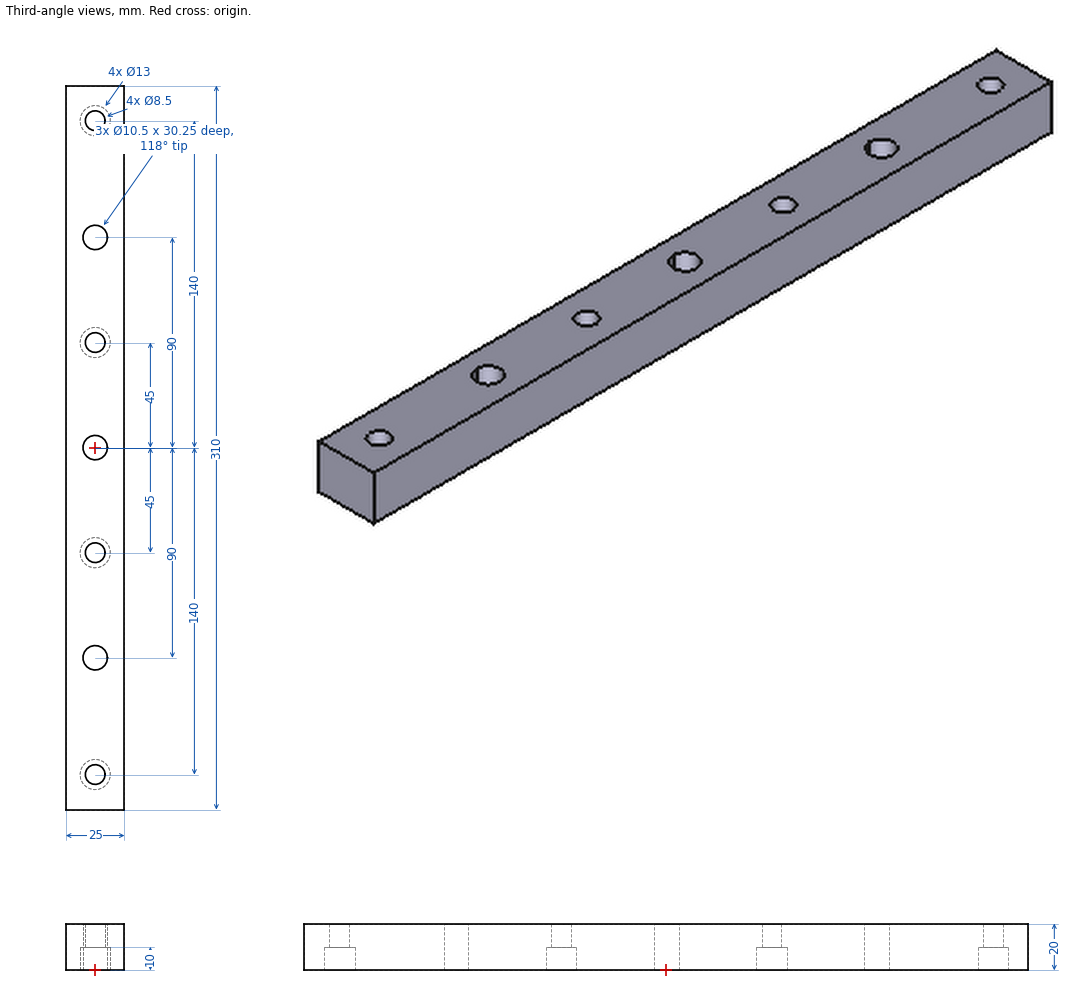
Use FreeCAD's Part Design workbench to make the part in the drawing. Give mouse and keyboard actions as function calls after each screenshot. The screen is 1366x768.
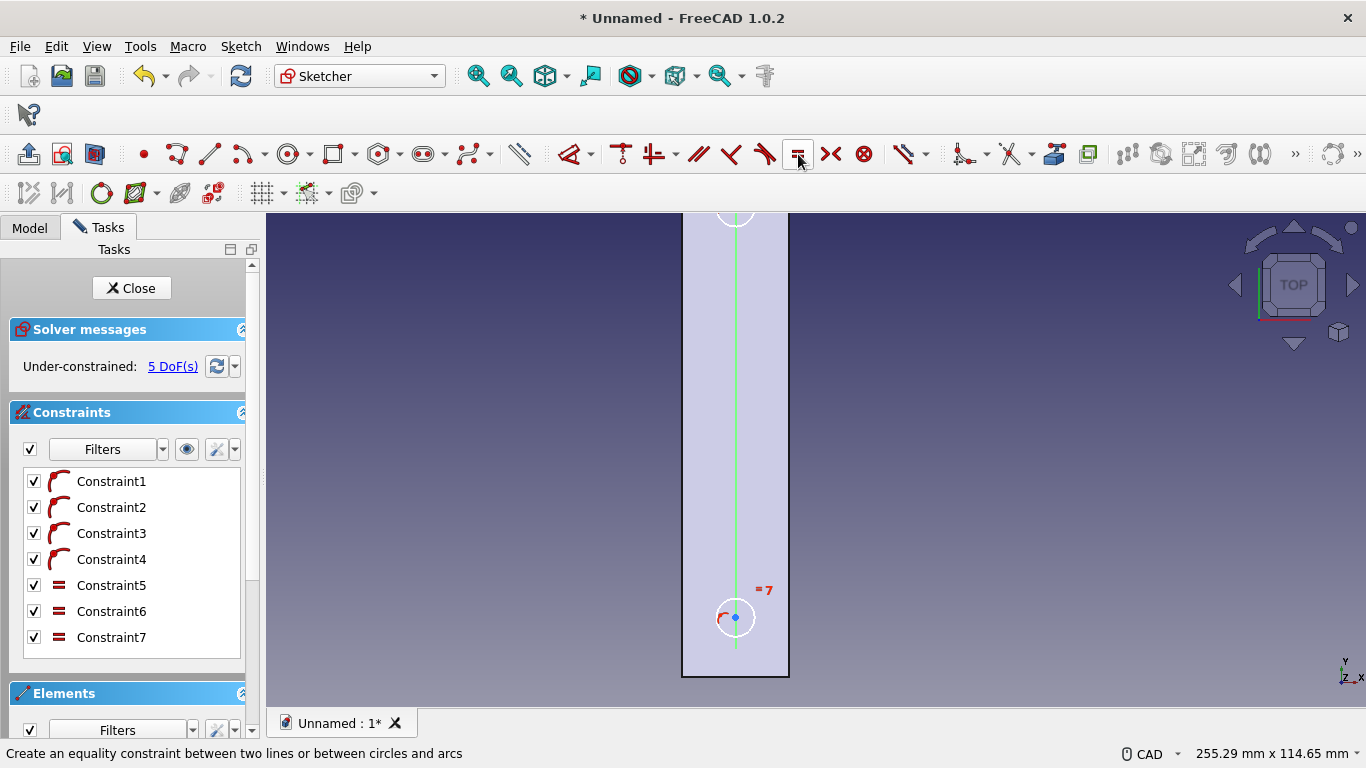
key(d)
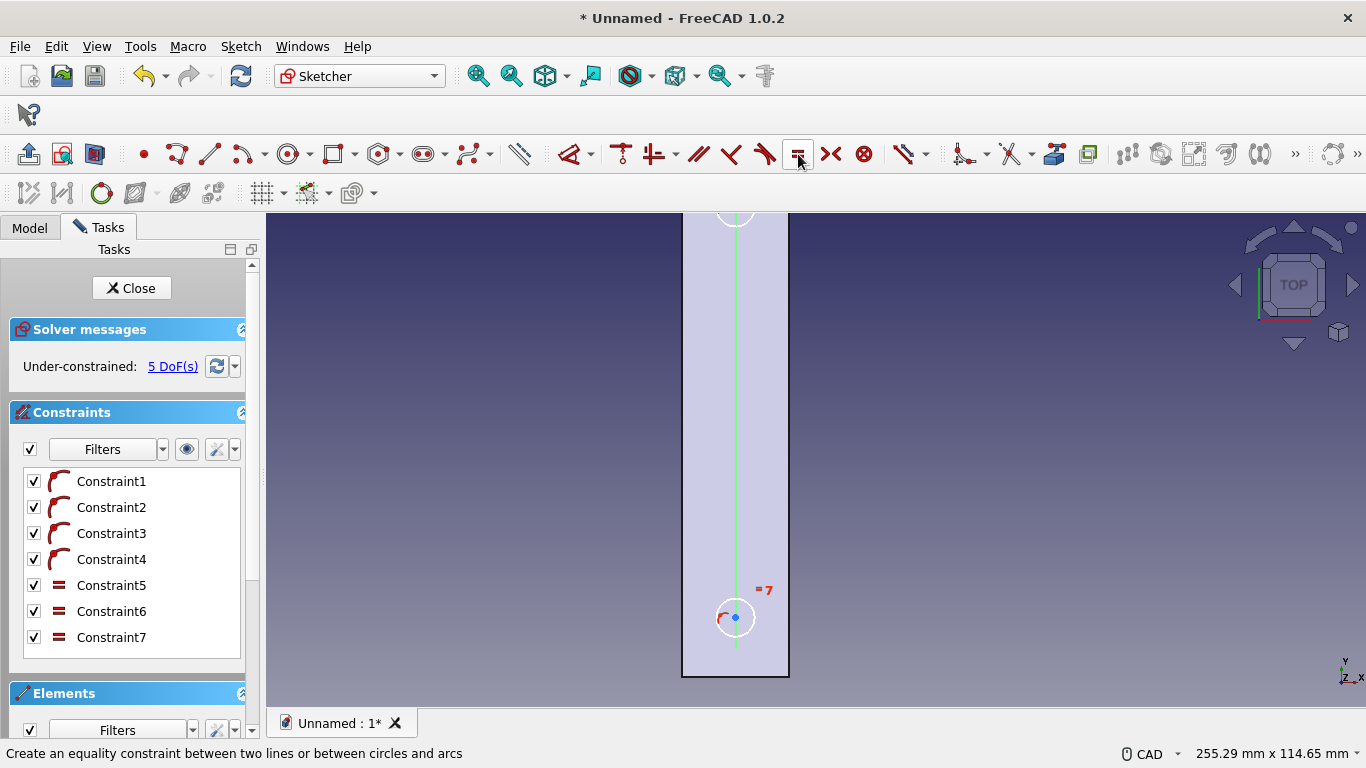
scroll(751, 607, down, 7)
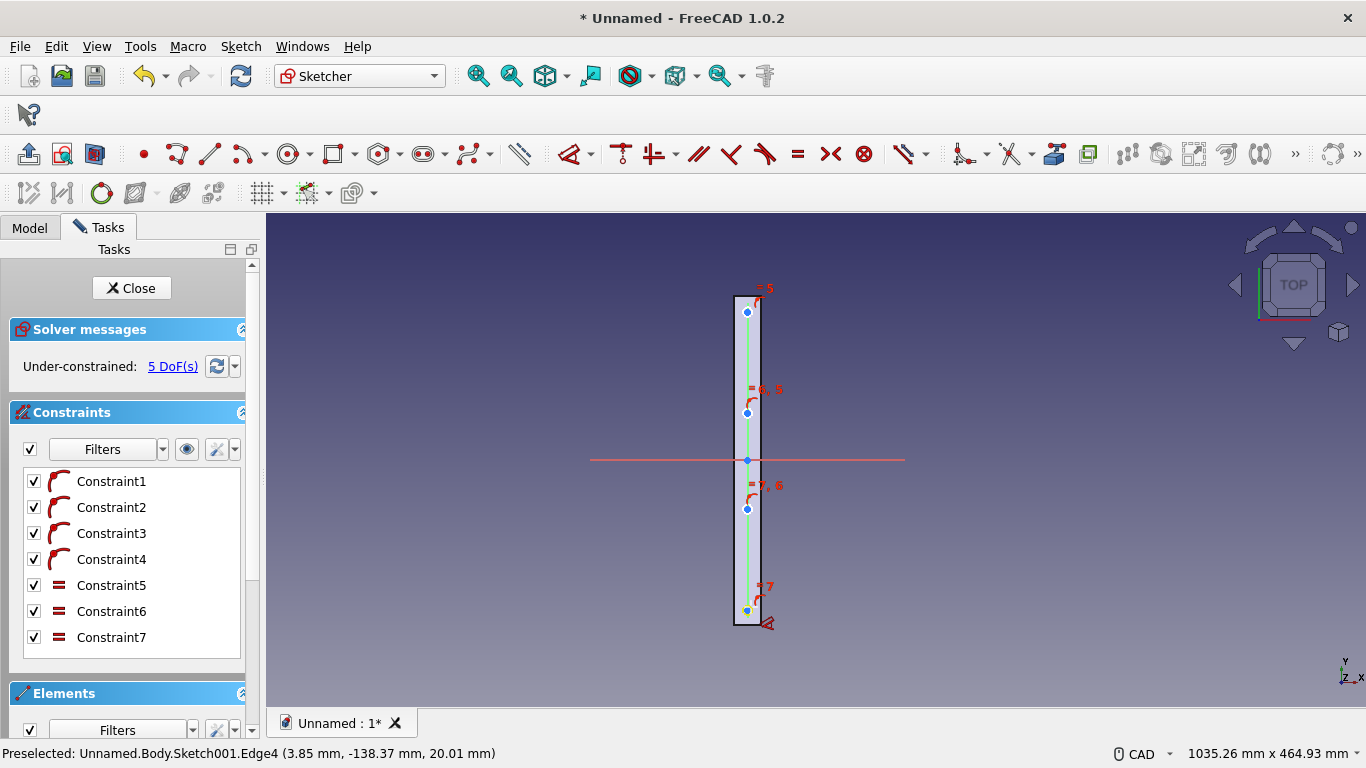
scroll(751, 309, up, 8)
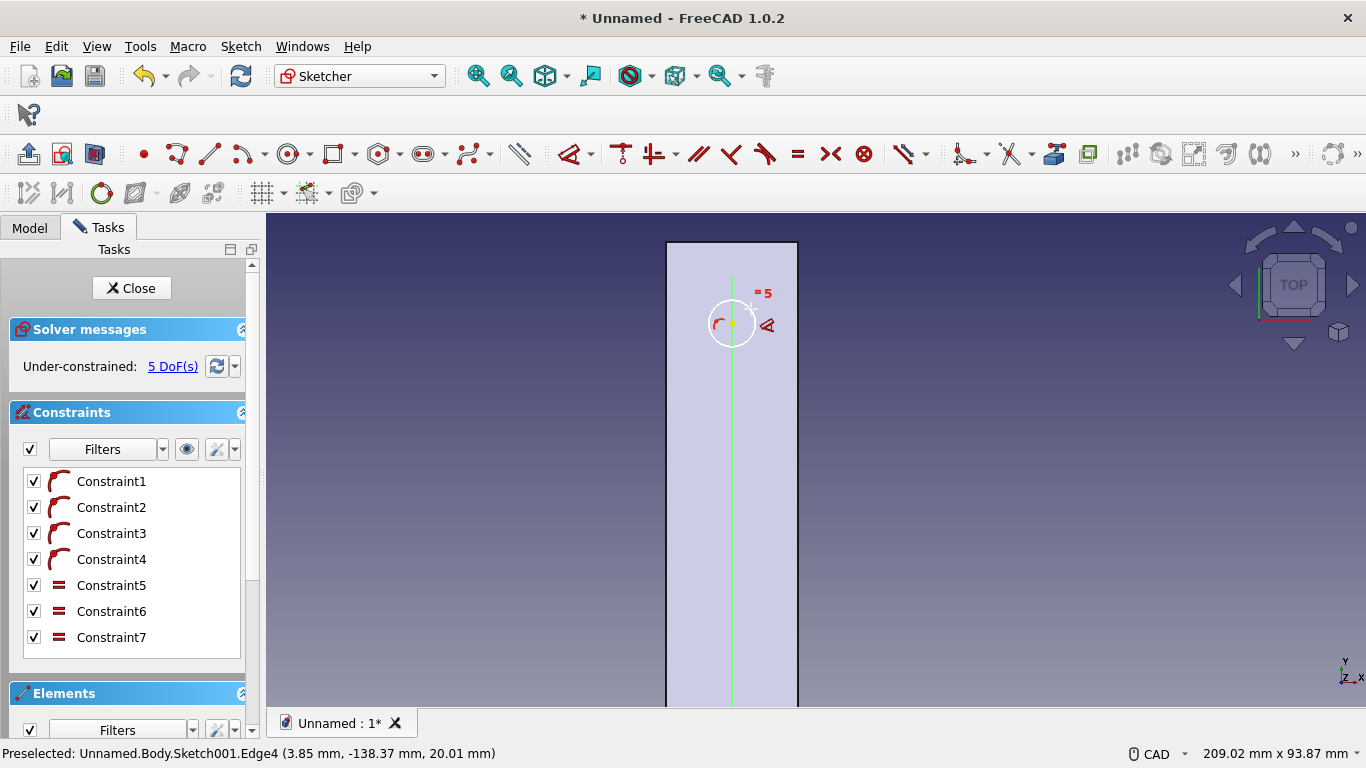
click(748, 307)
click(770, 284)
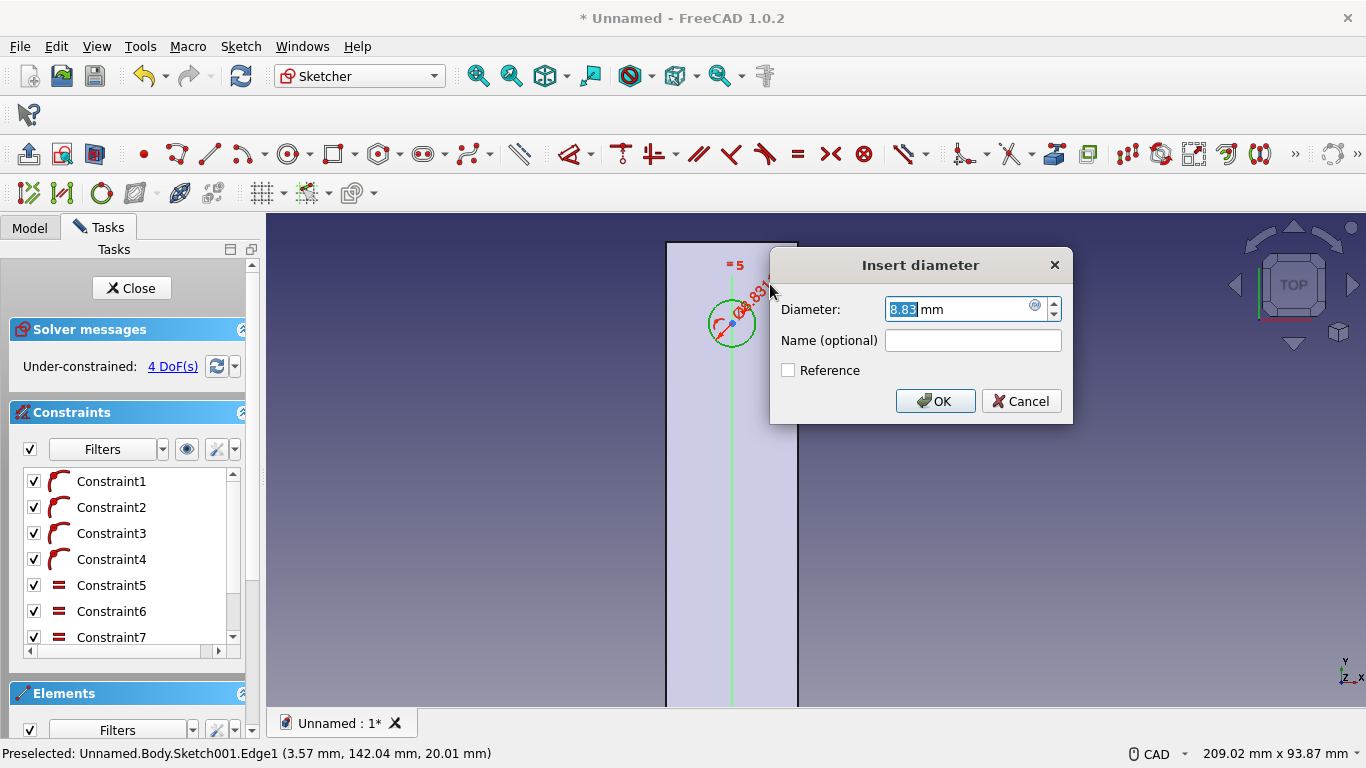
text(8.5)
key(Return)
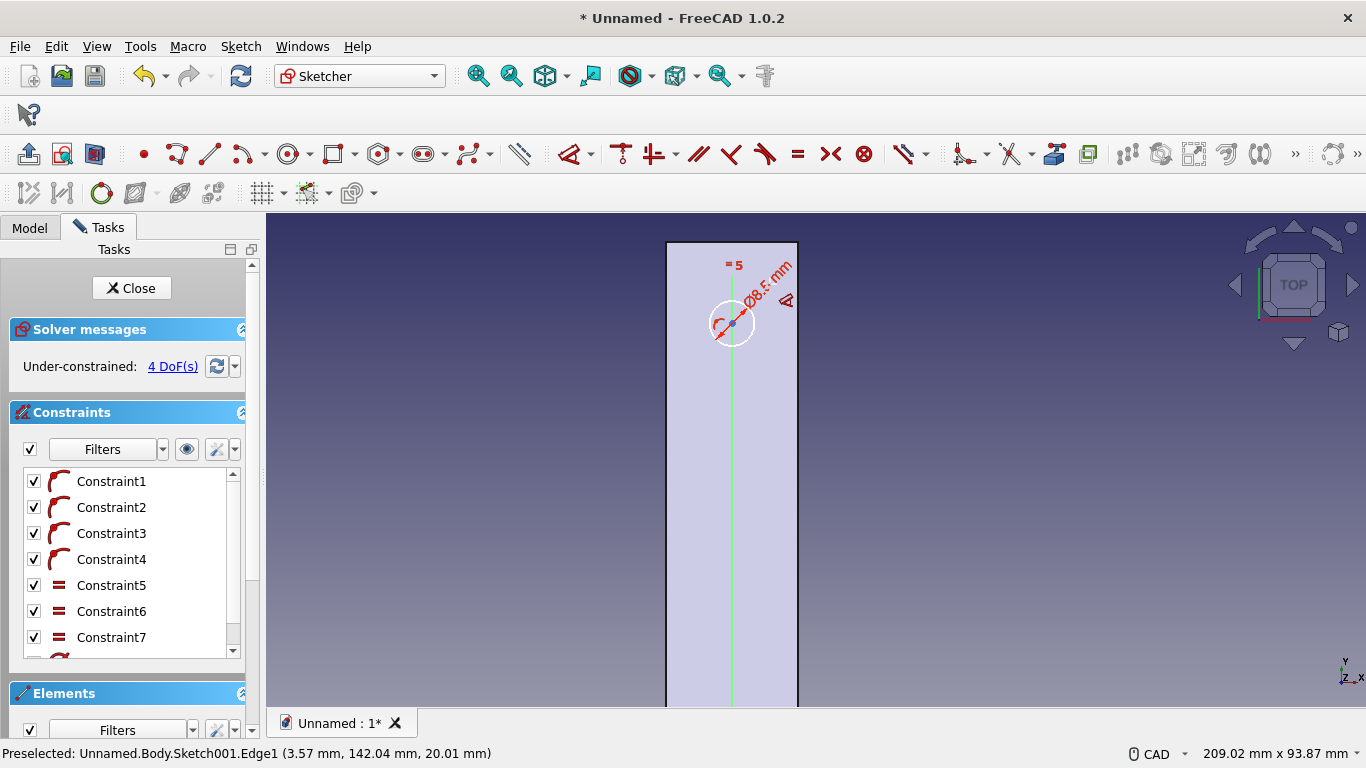
scroll(751, 309, down, 8)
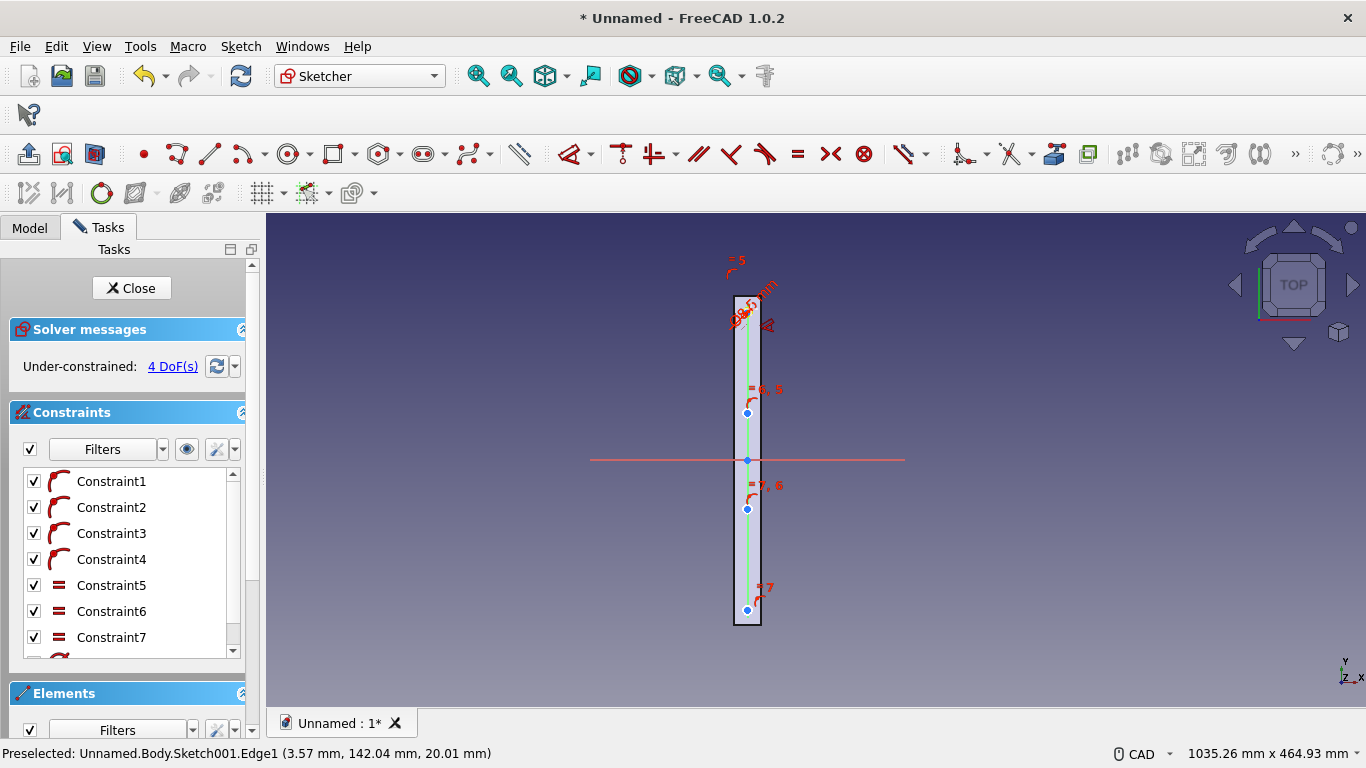
click(748, 413)
click(782, 437)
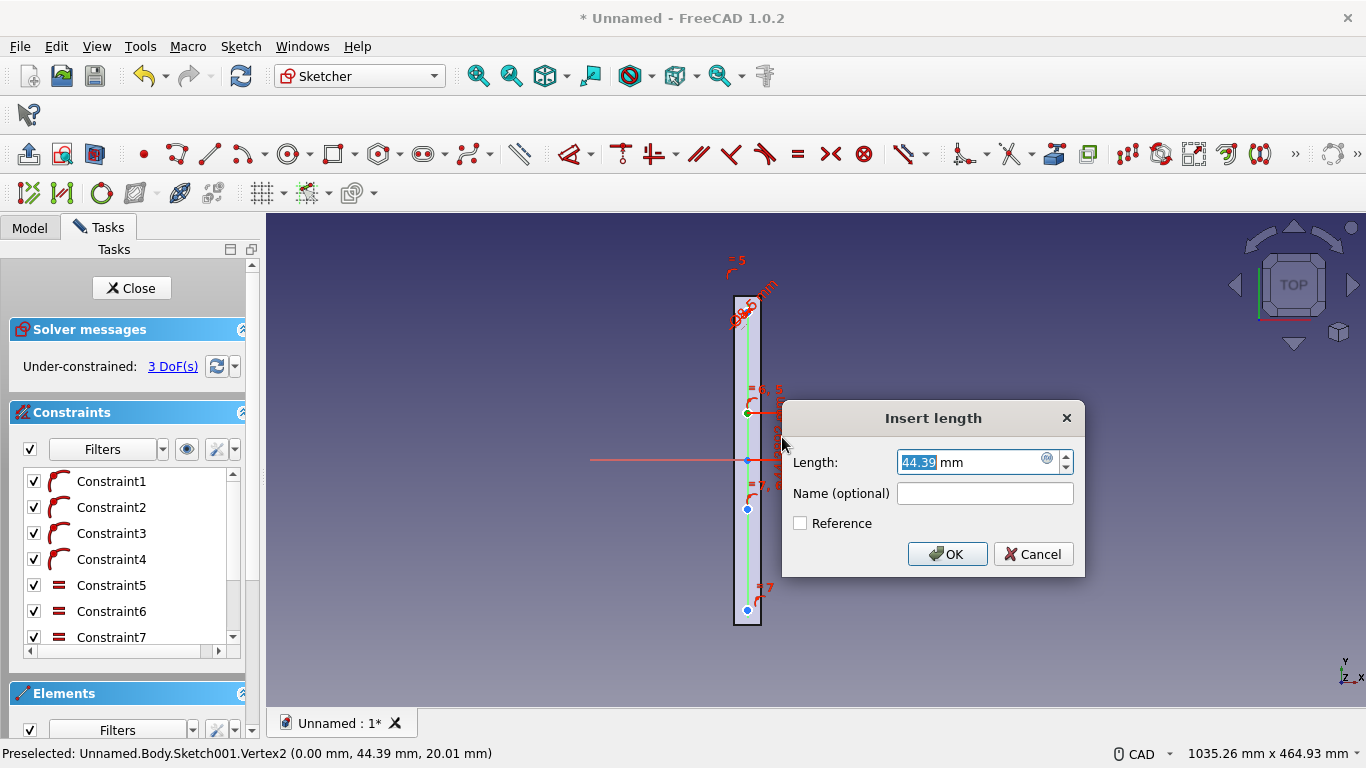
text(45)
key(Return)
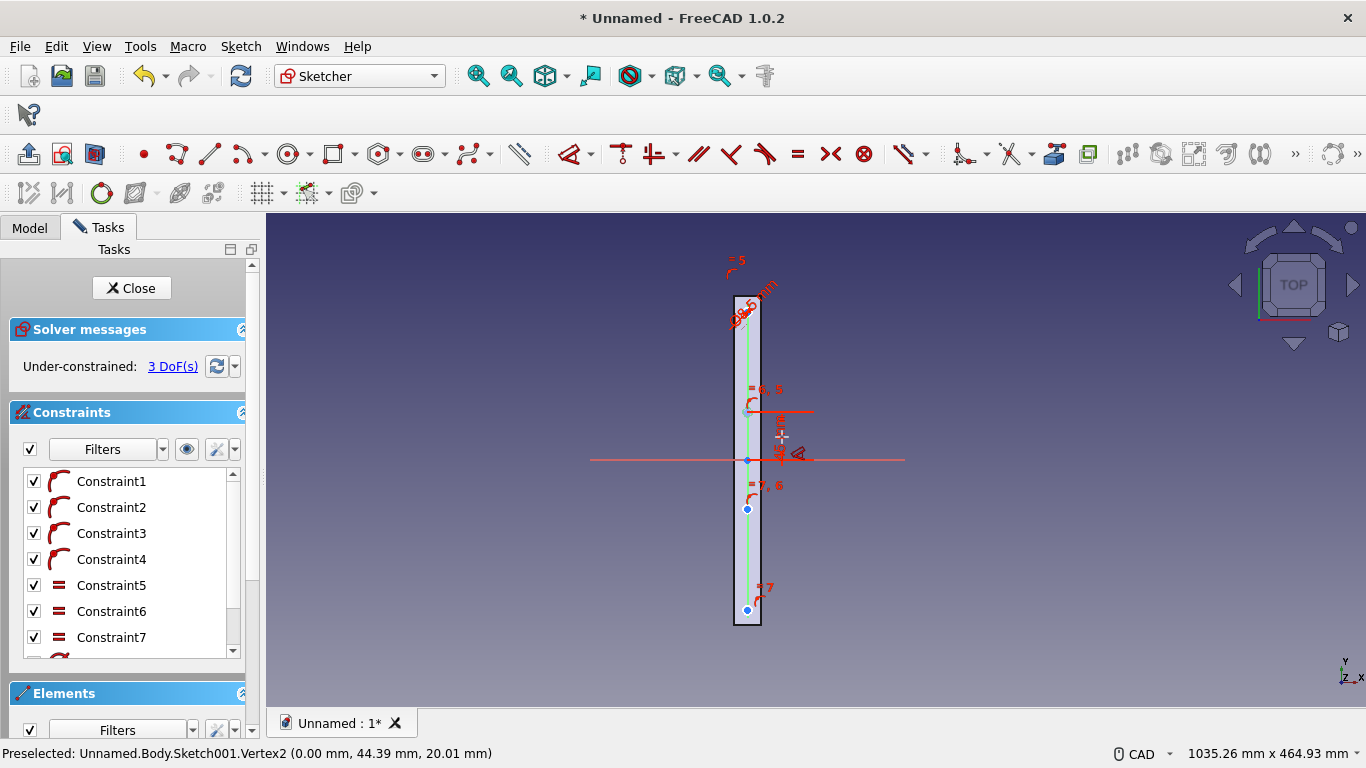
click(748, 509)
click(782, 485)